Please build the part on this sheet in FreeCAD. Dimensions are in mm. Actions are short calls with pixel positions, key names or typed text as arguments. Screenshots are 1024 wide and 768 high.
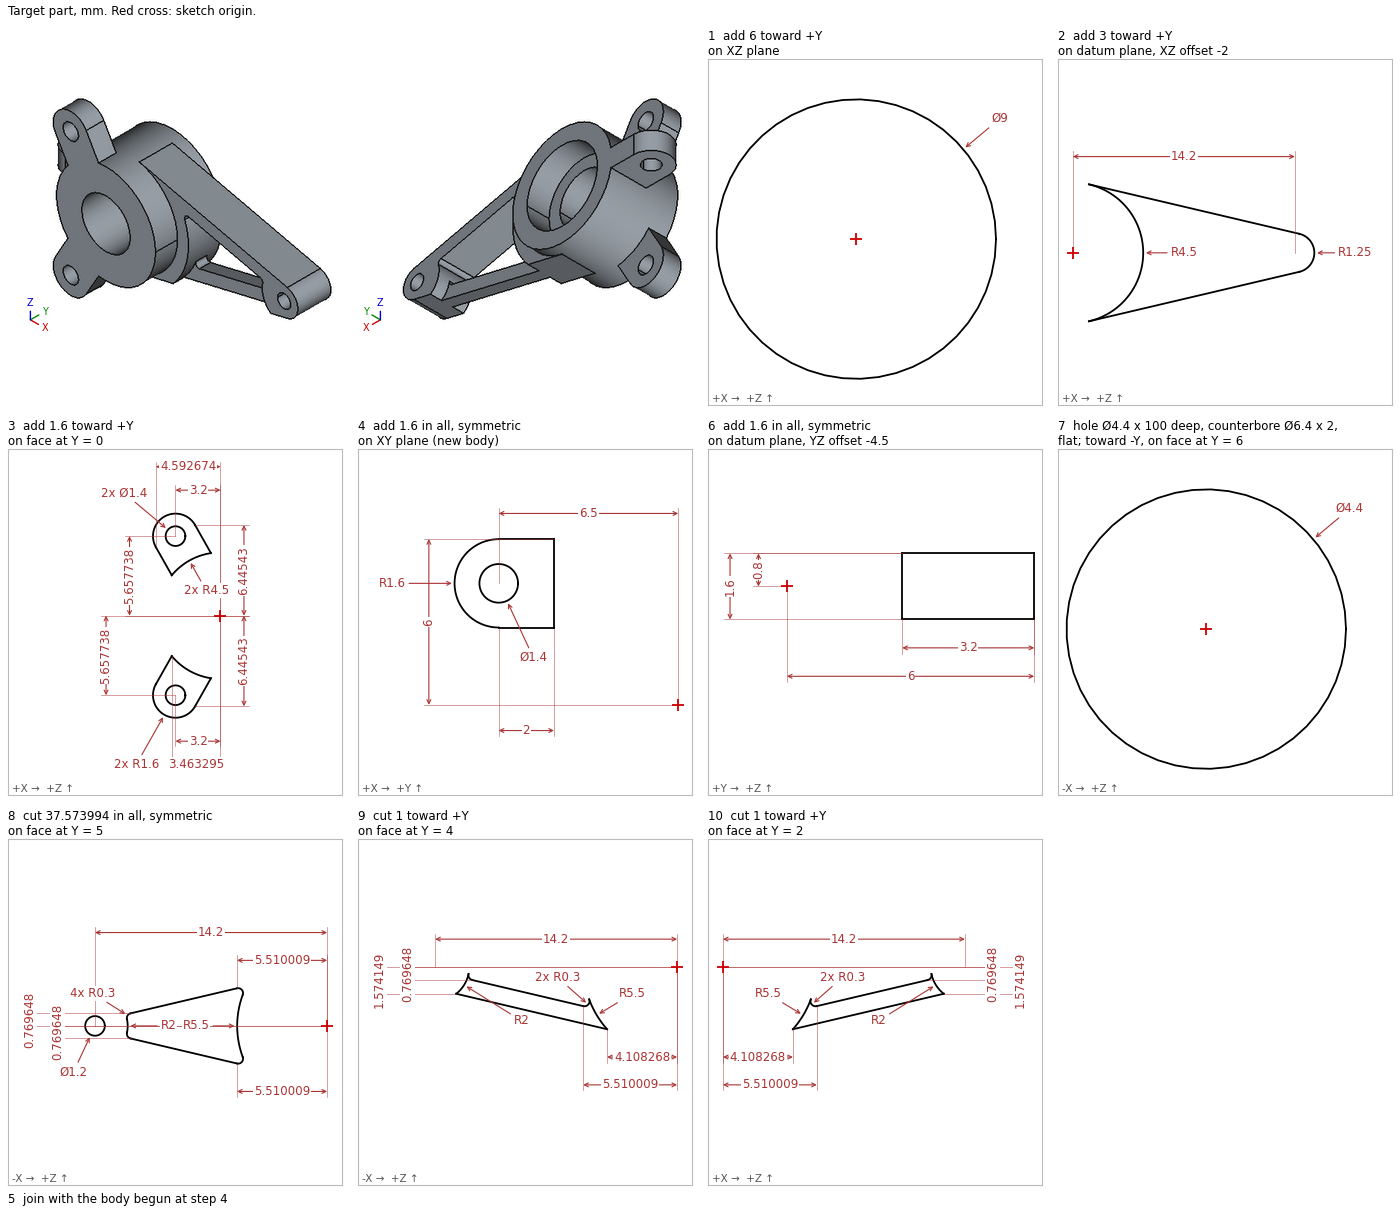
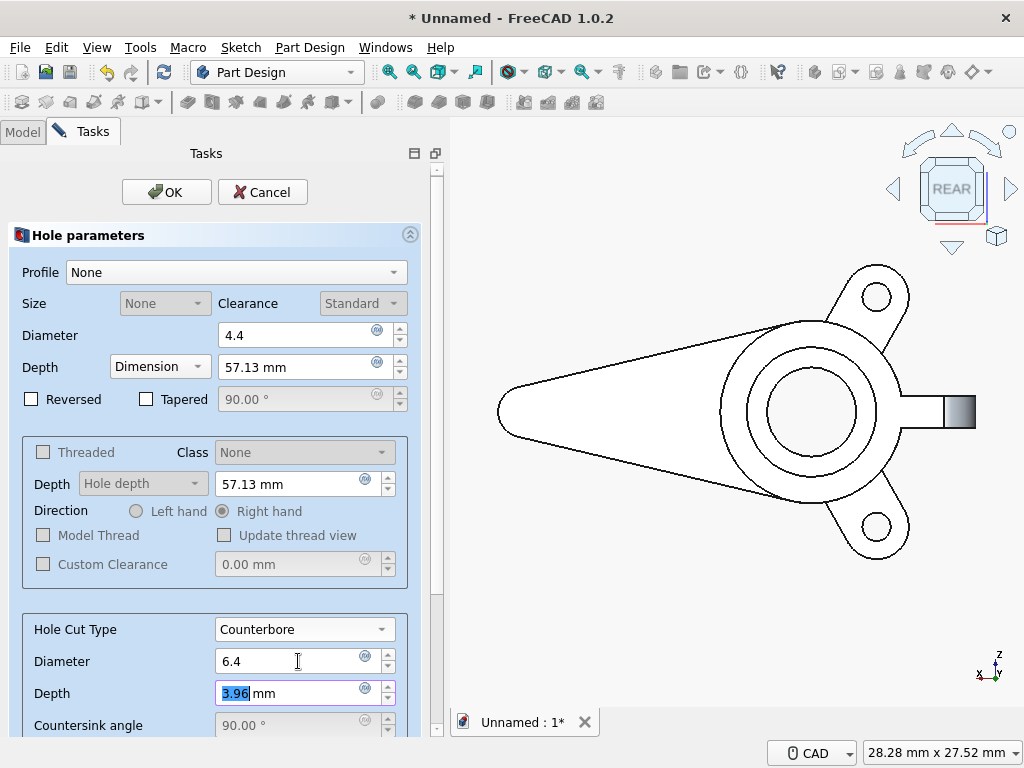
text(2)
key(Tab)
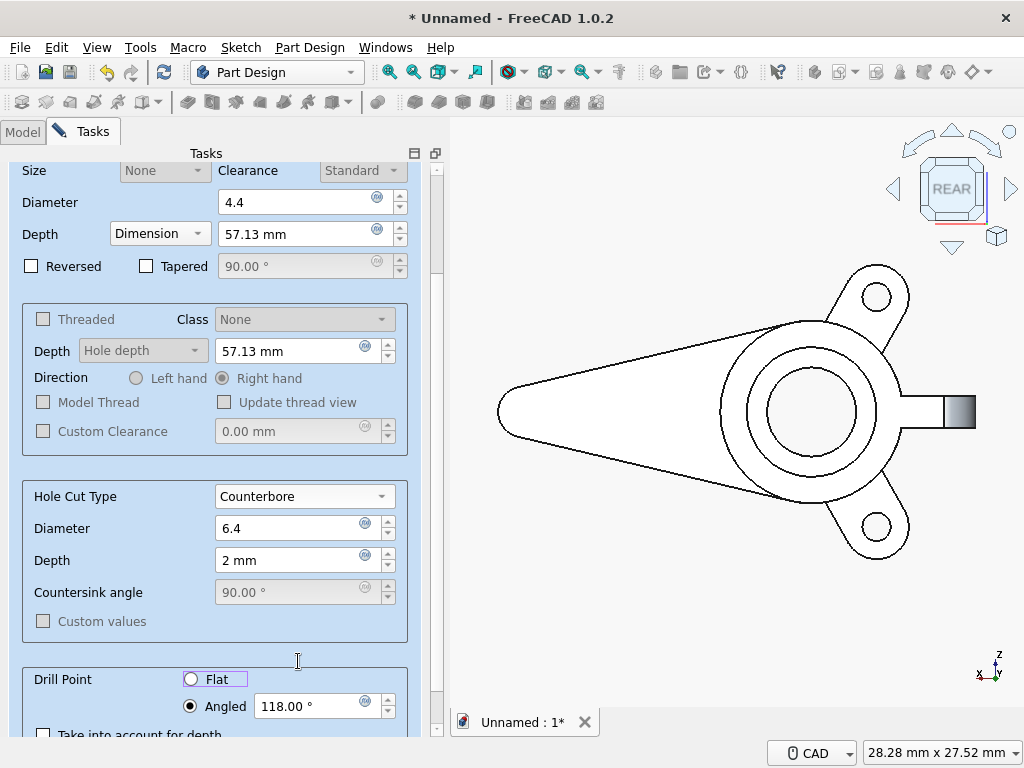
click(191, 679)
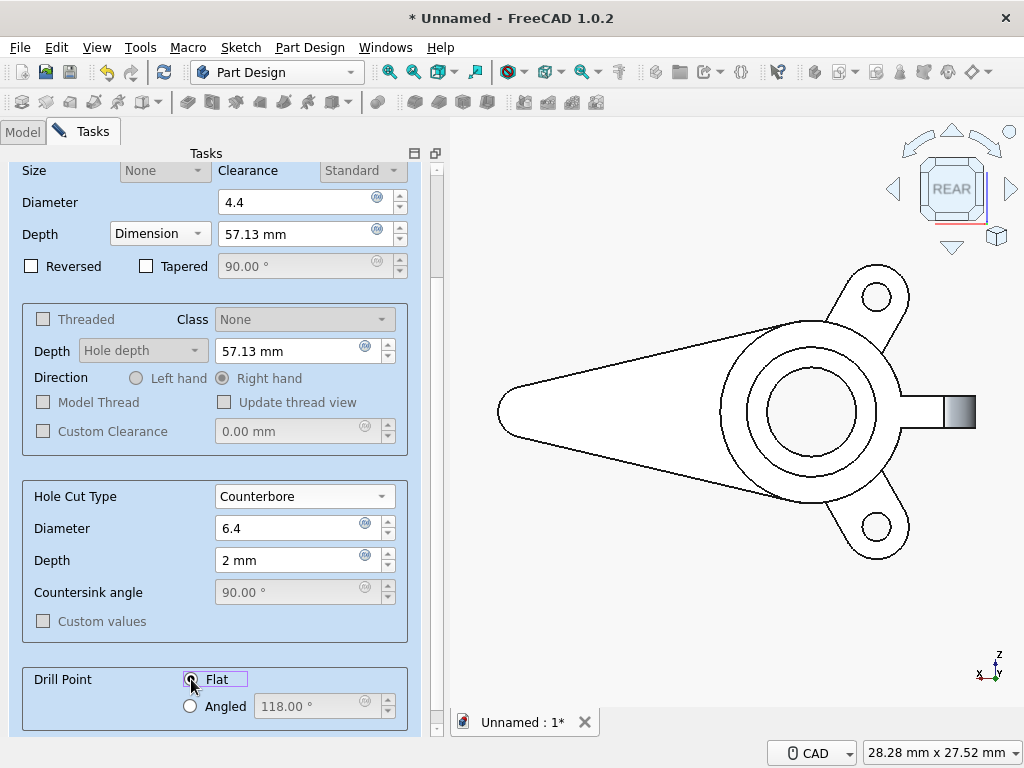
scroll(437, 450, up, 3)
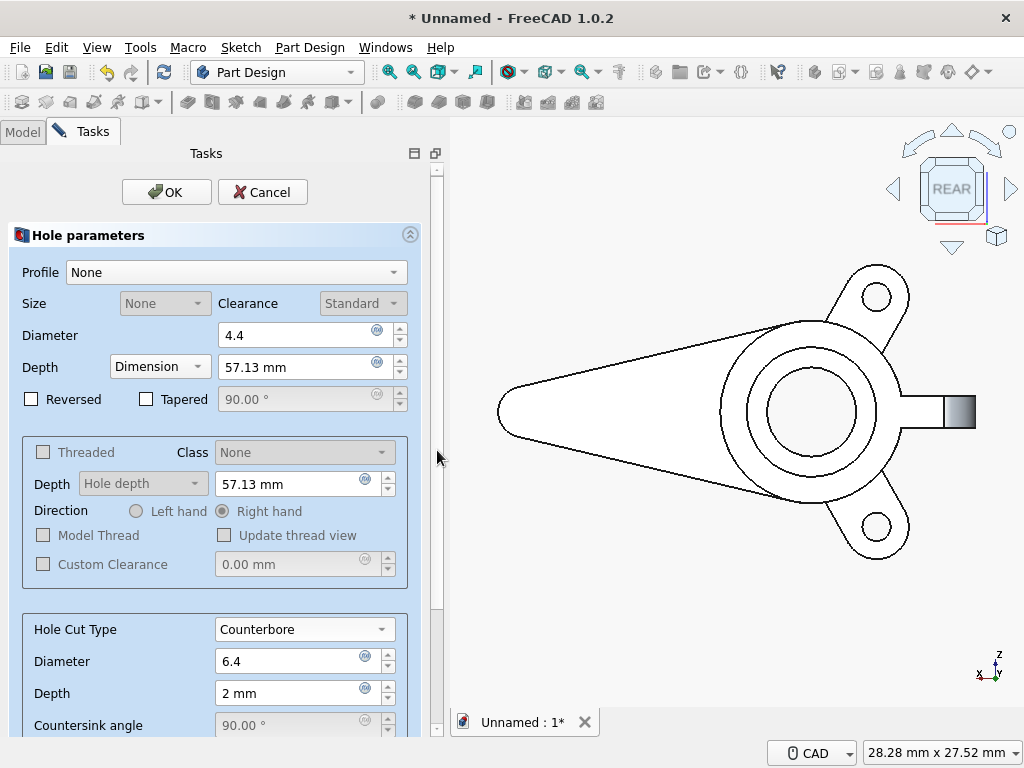
click(167, 192)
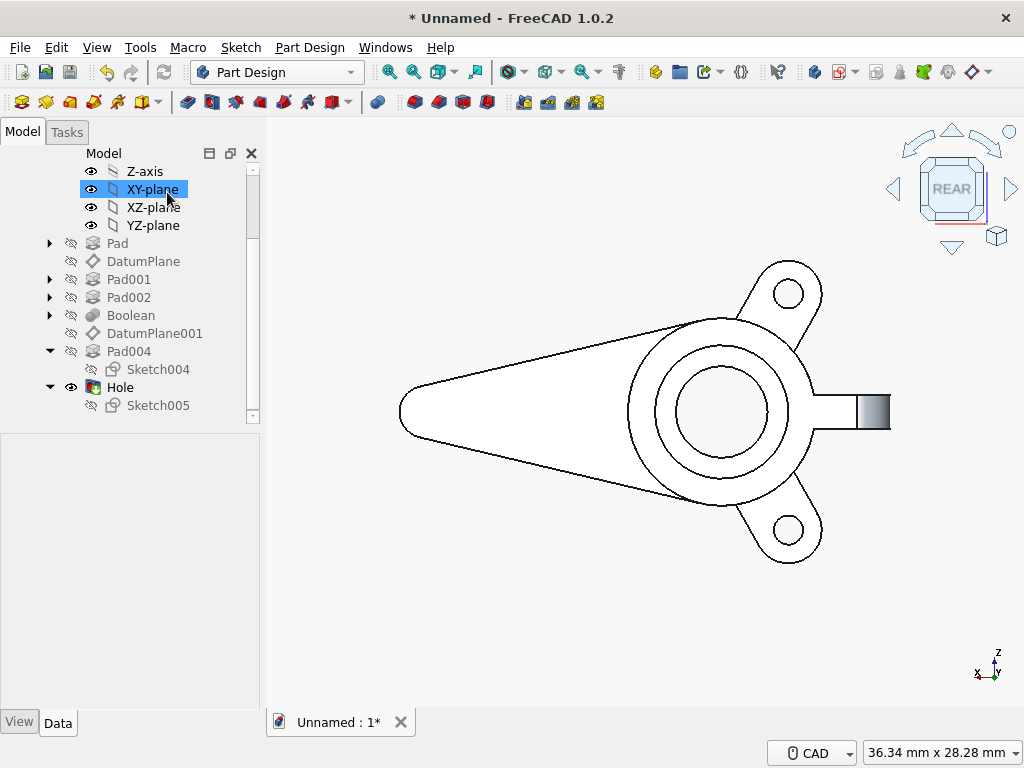
click(550, 411)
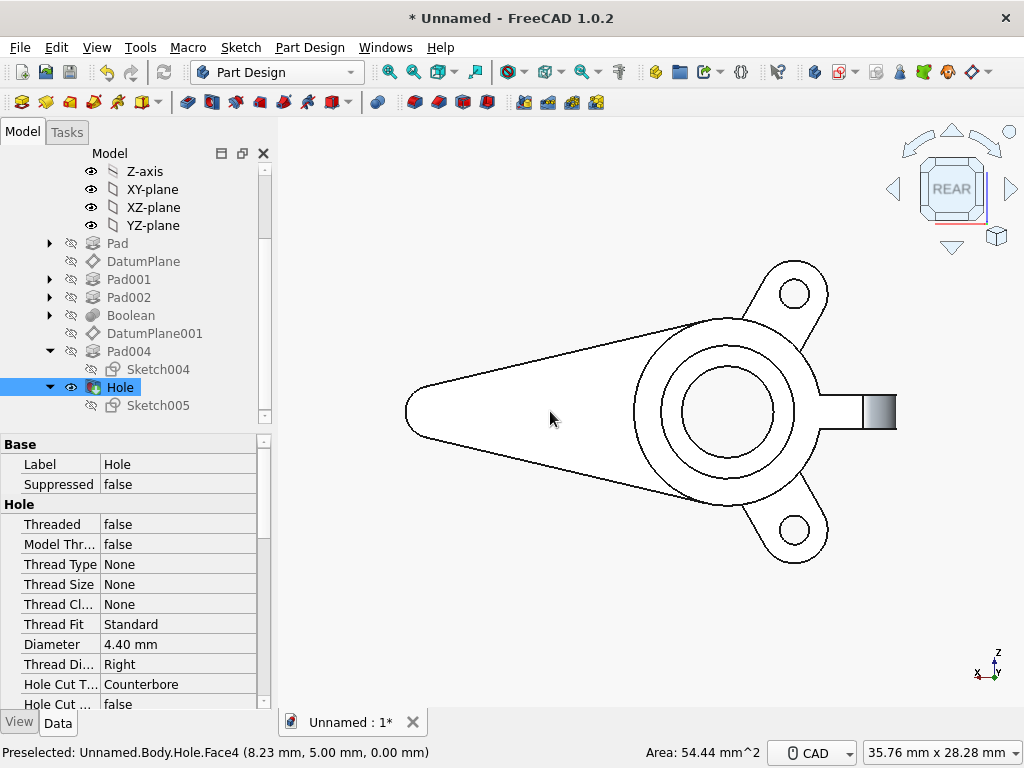
click(840, 72)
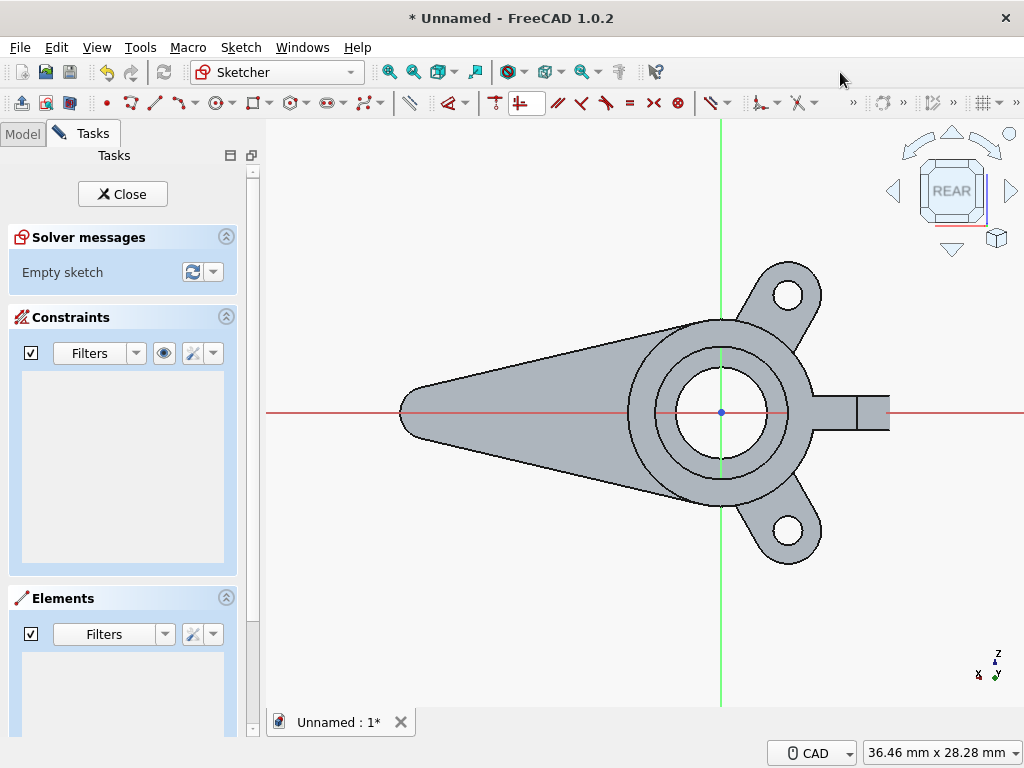
click(70, 104)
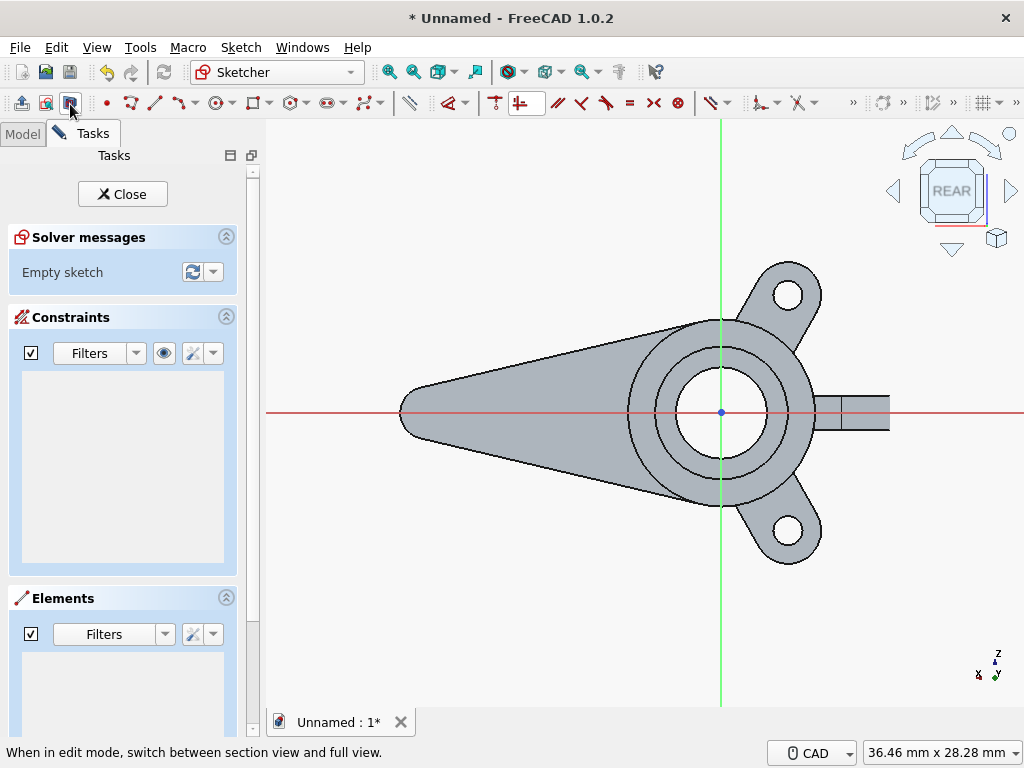
key(g)
key(l)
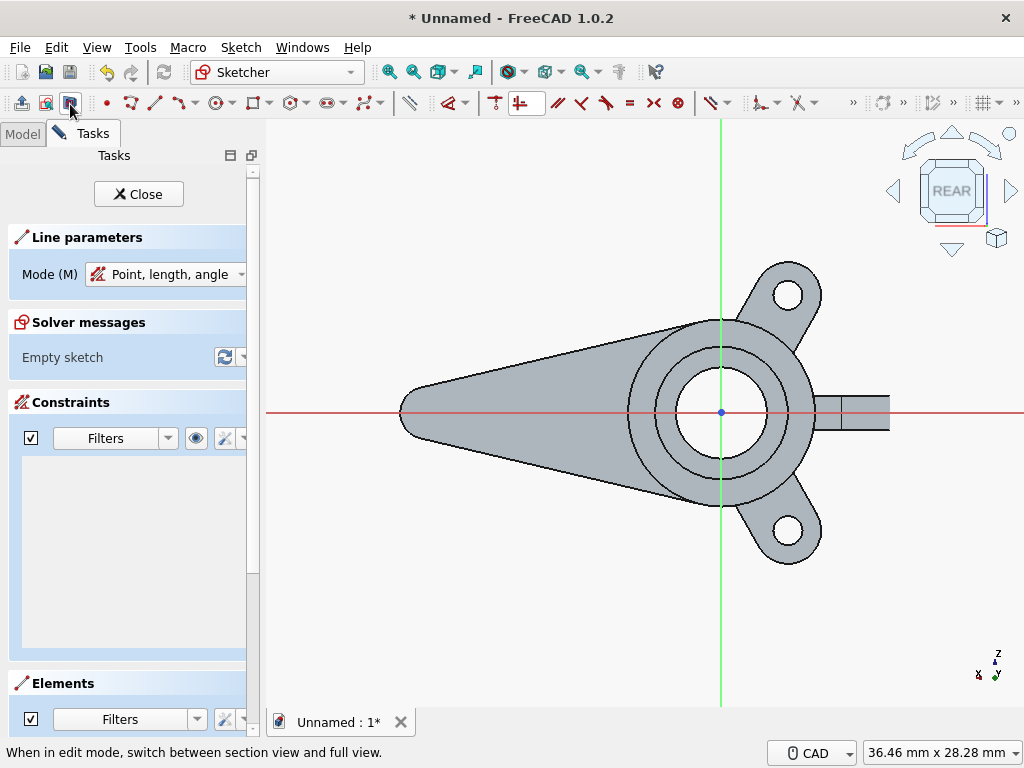
click(472, 429)
click(607, 461)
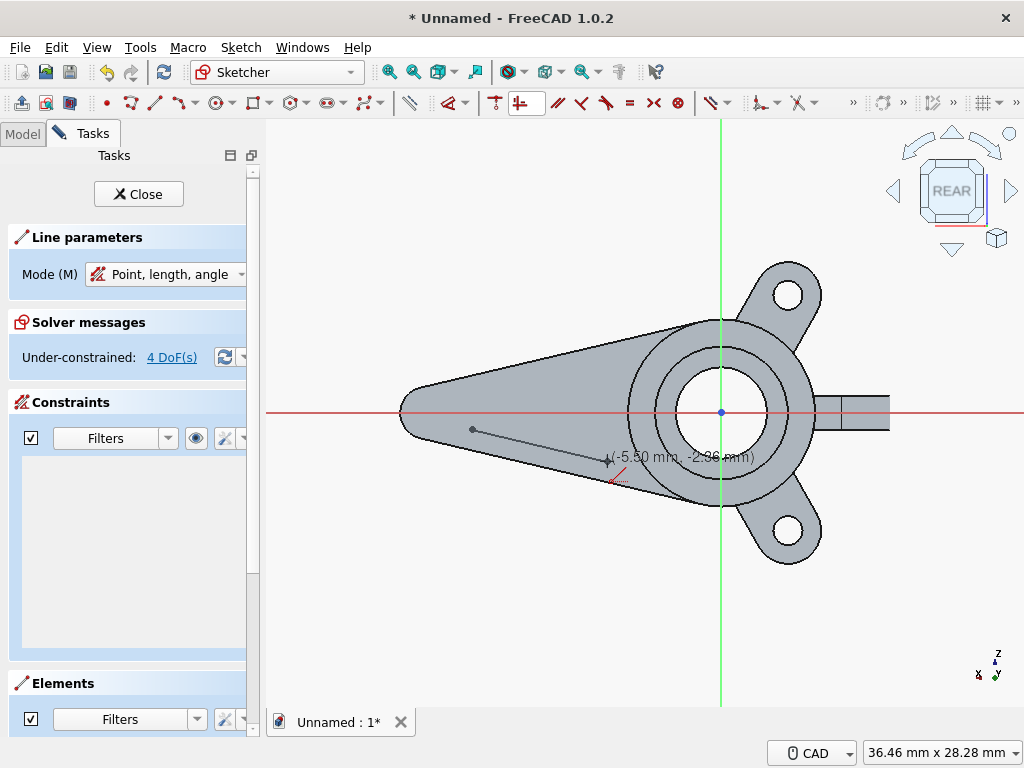
click(607, 365)
click(472, 397)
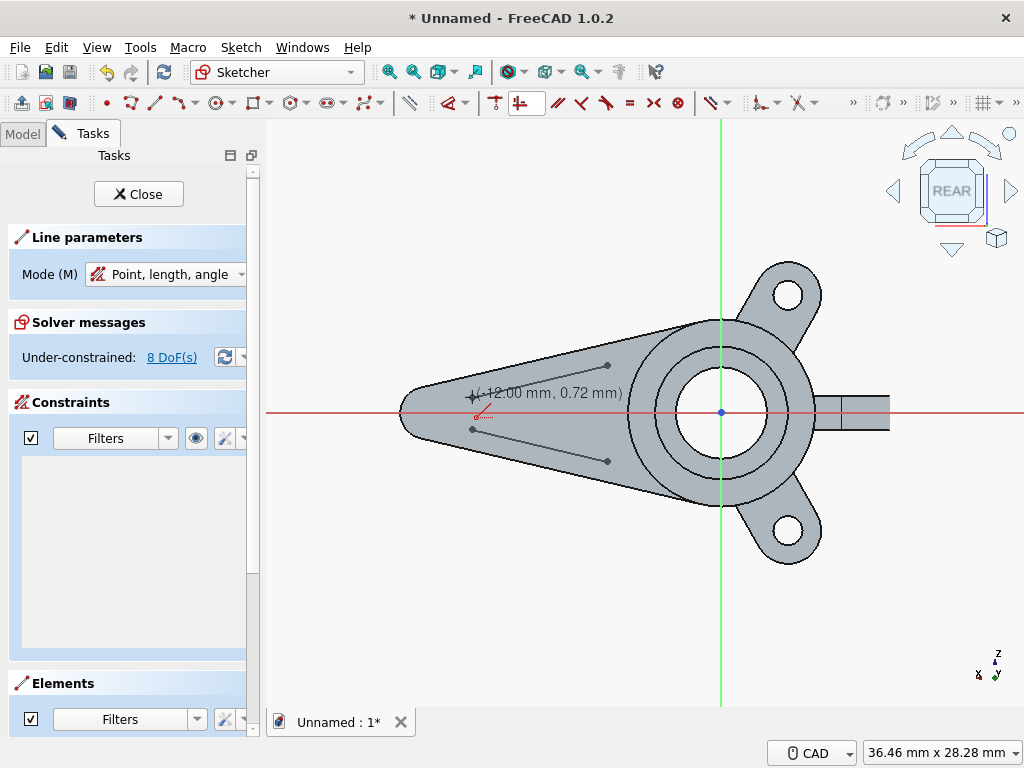
key(g)
key(3)
key(a)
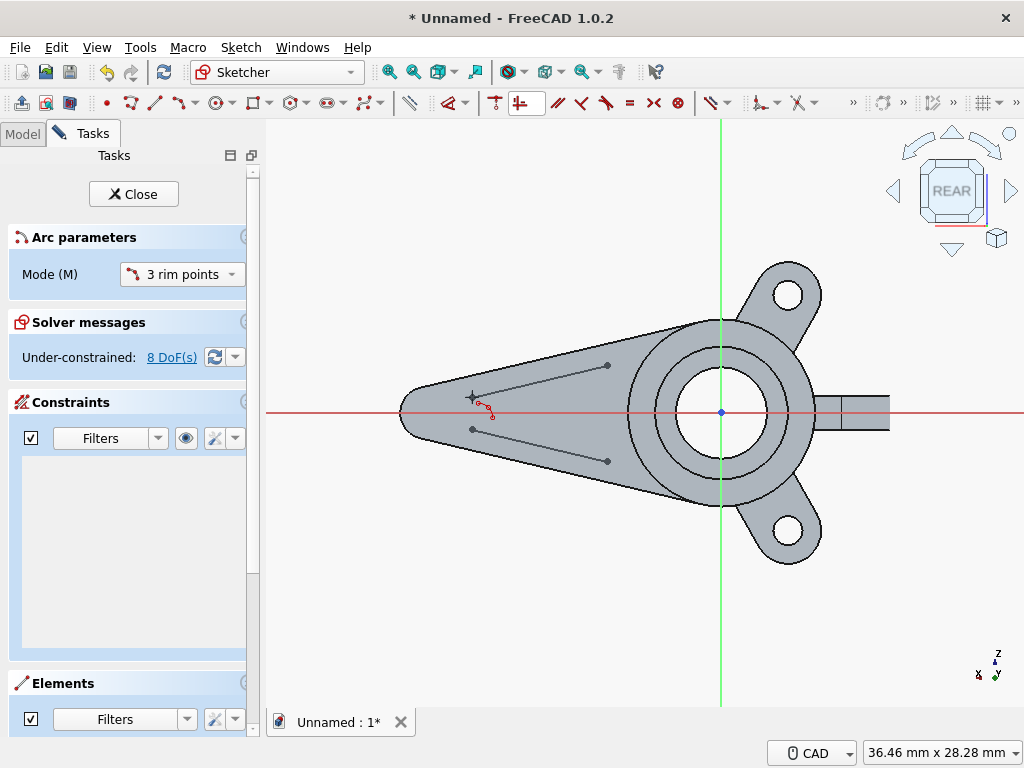
click(607, 462)